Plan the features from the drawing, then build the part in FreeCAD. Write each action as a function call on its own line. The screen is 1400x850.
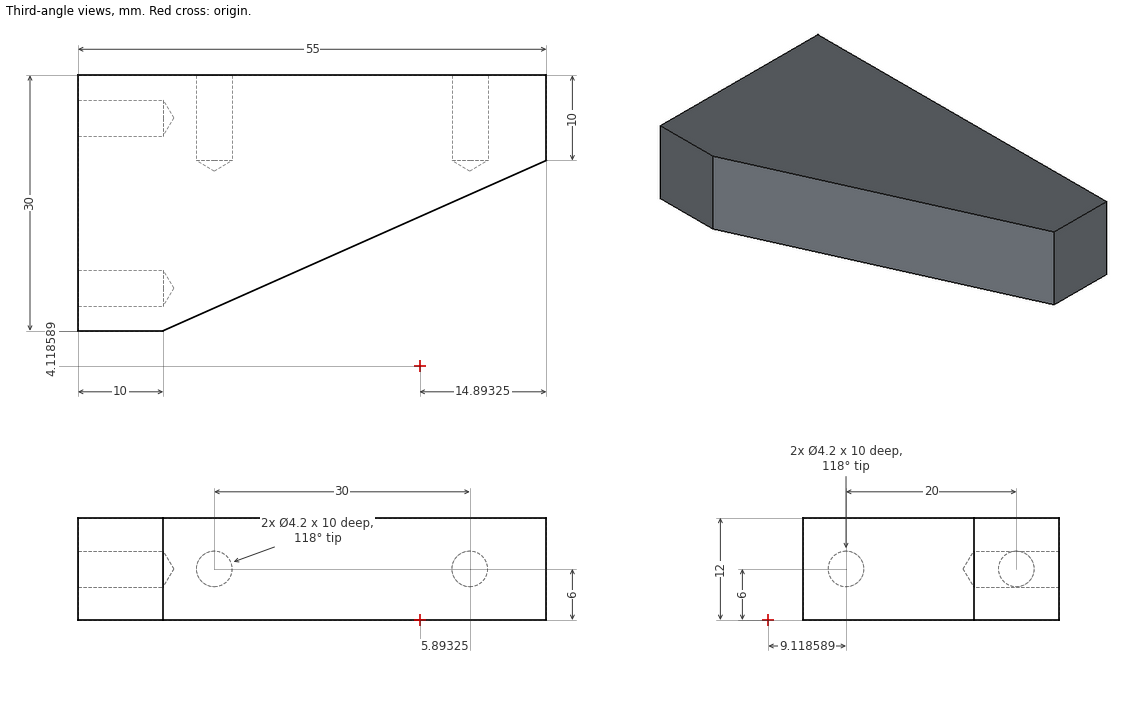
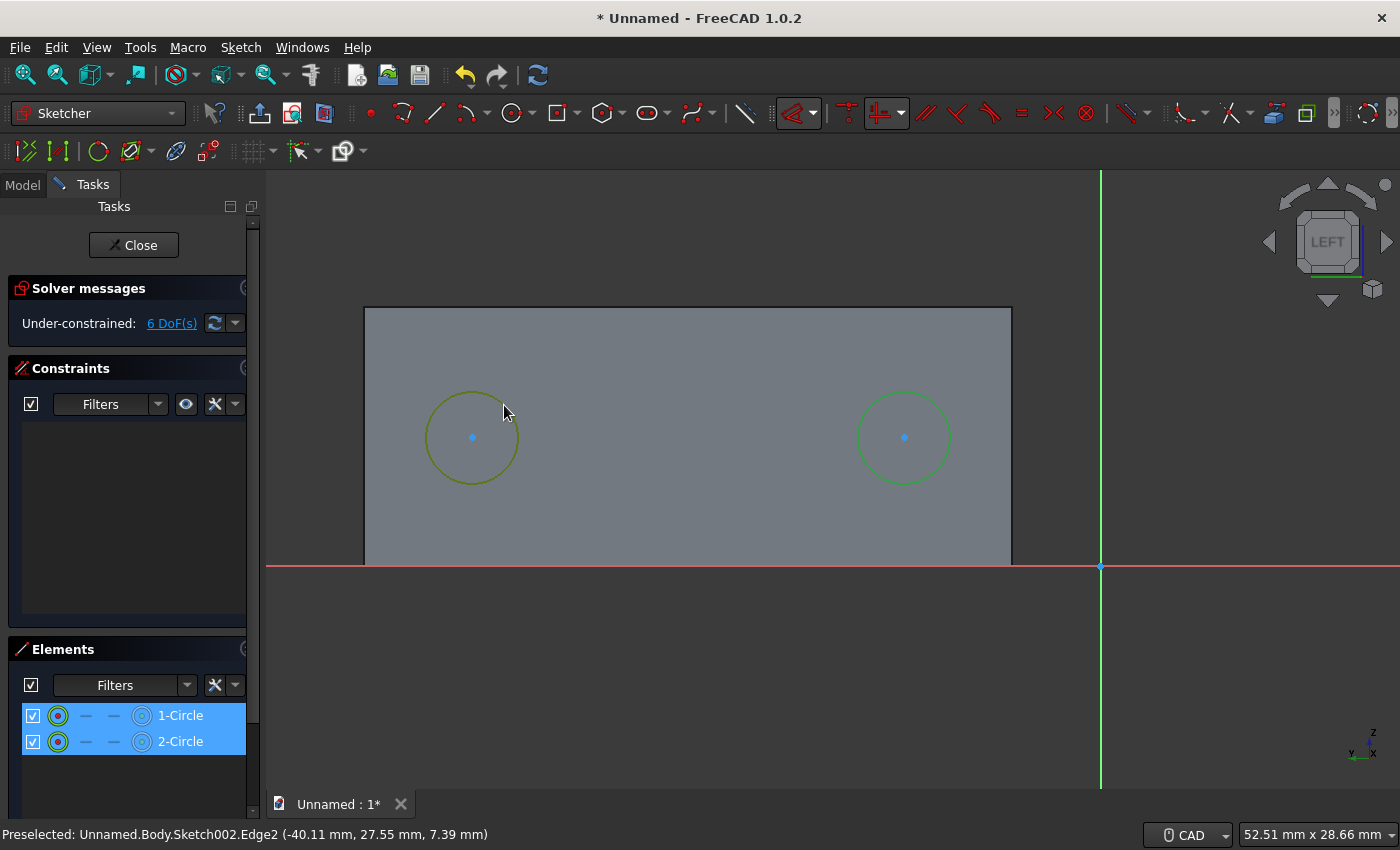
key(e)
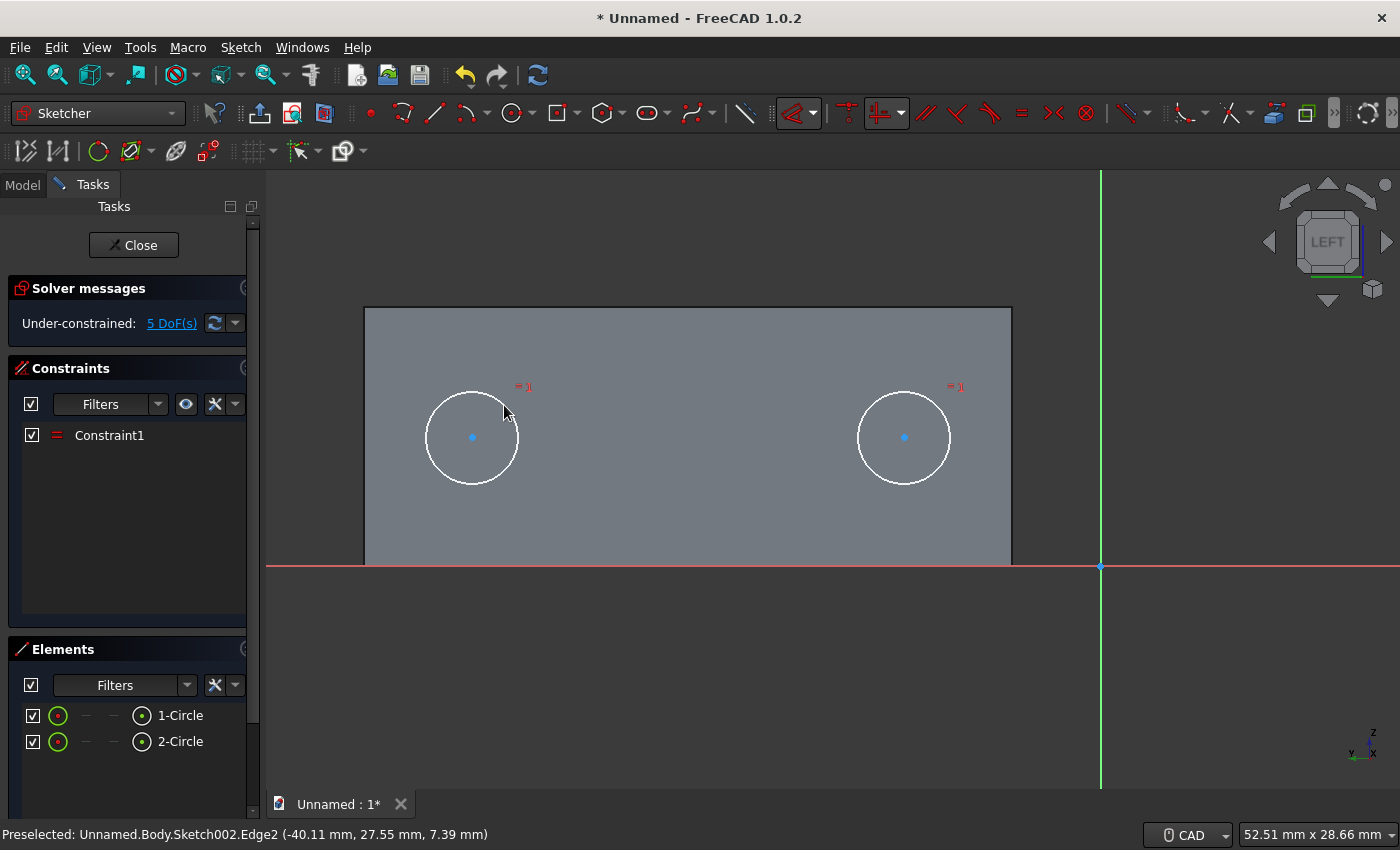
click(936, 405)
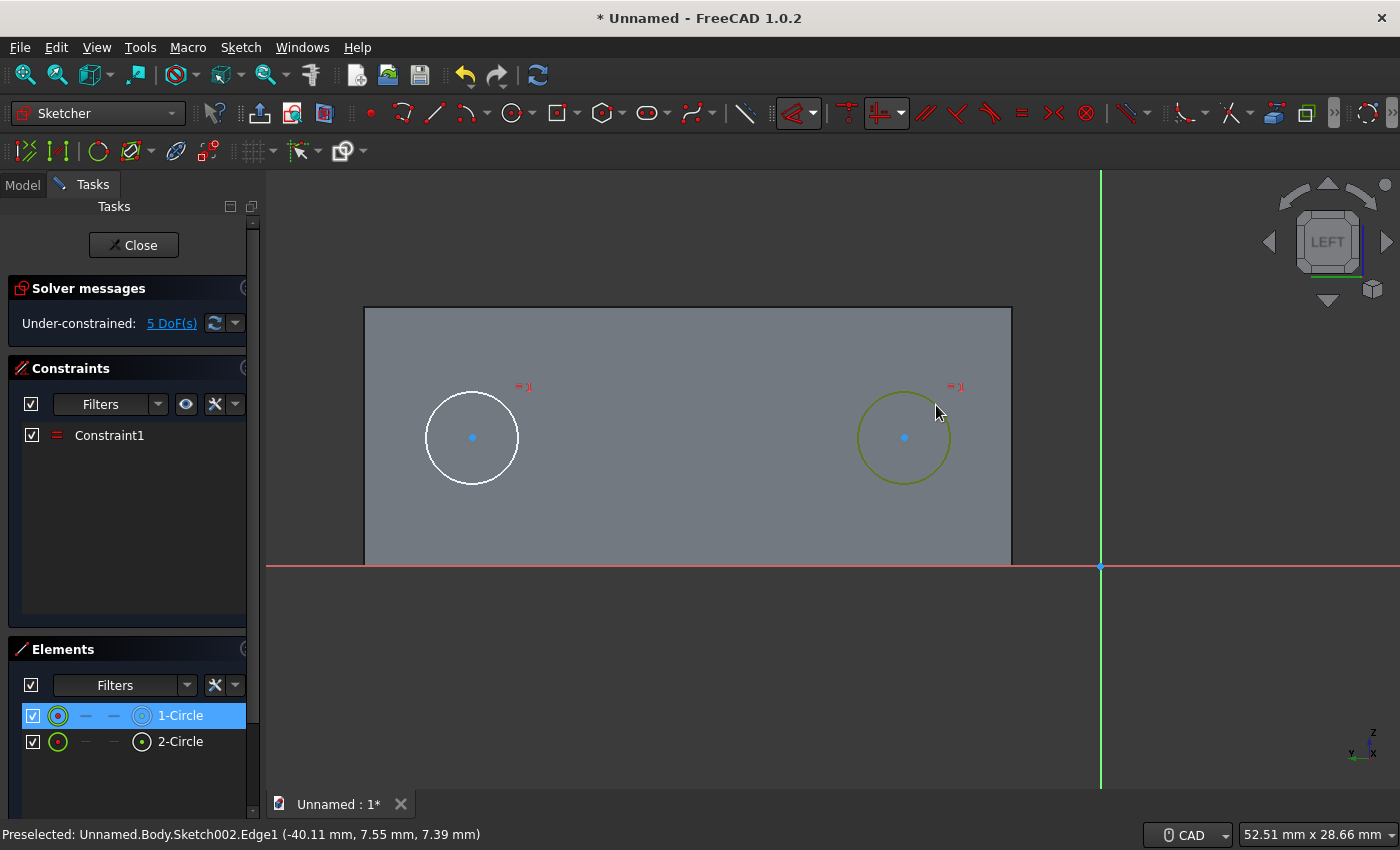
click(816, 114)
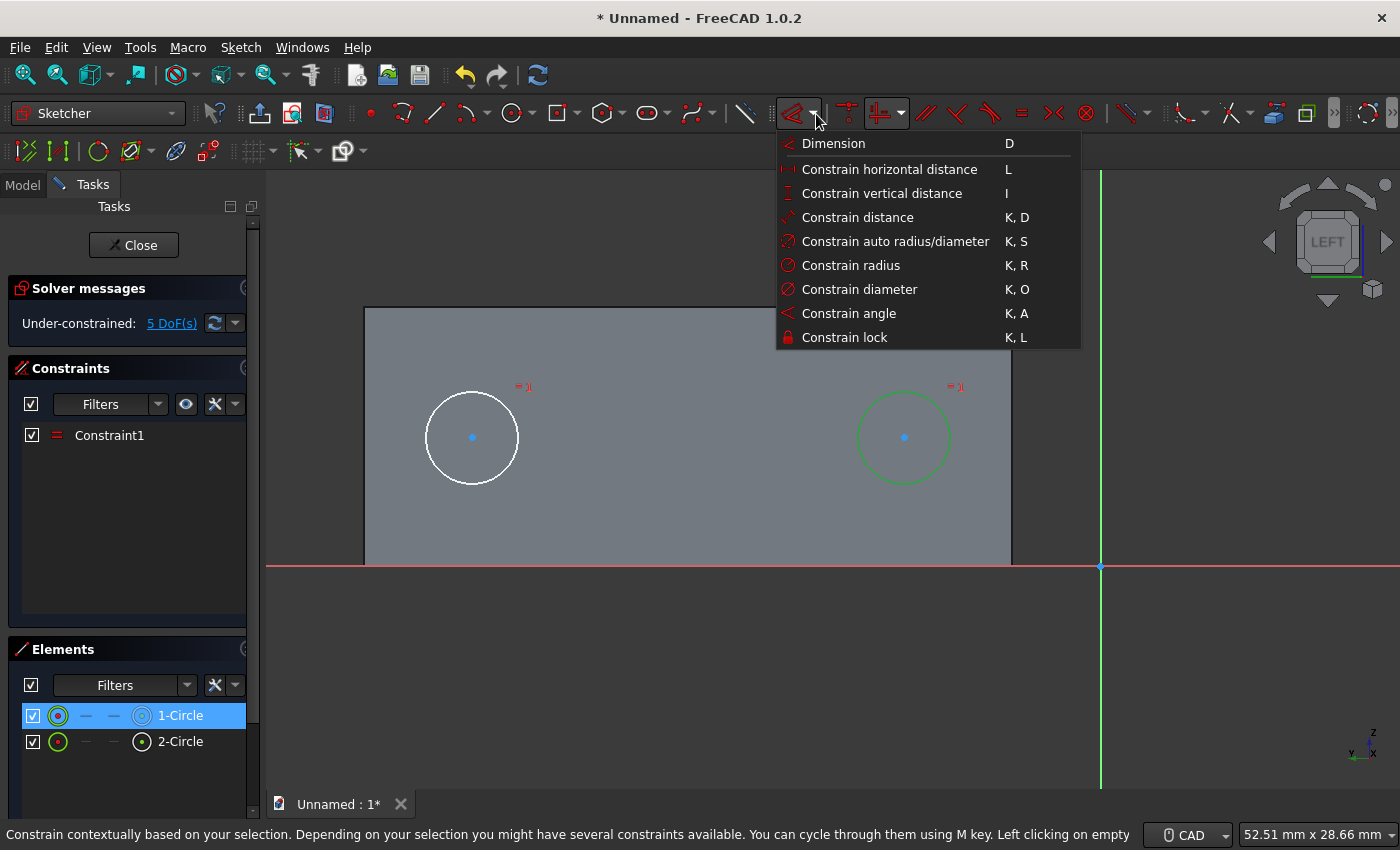
click(929, 289)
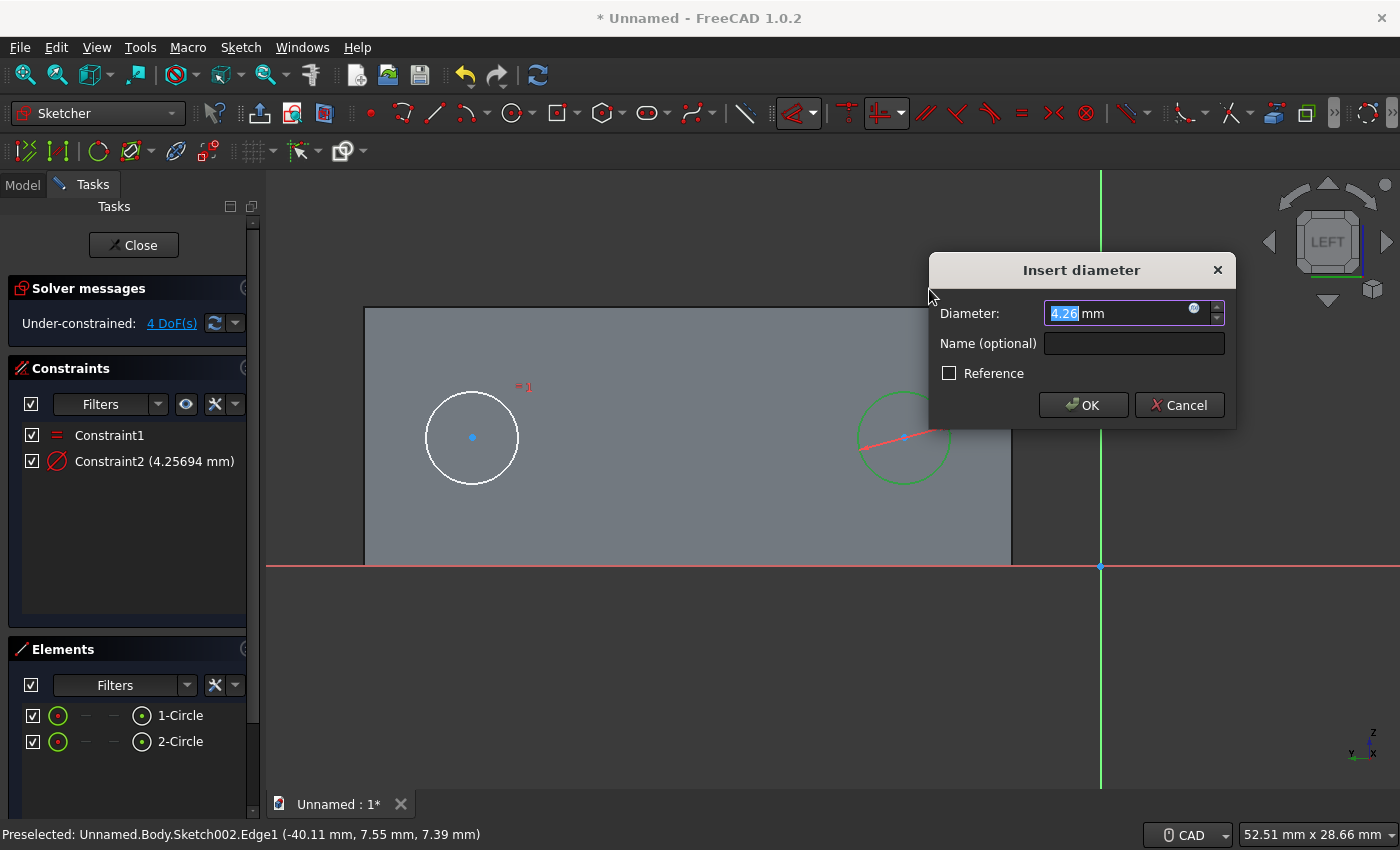
text(4.2)
key(Return)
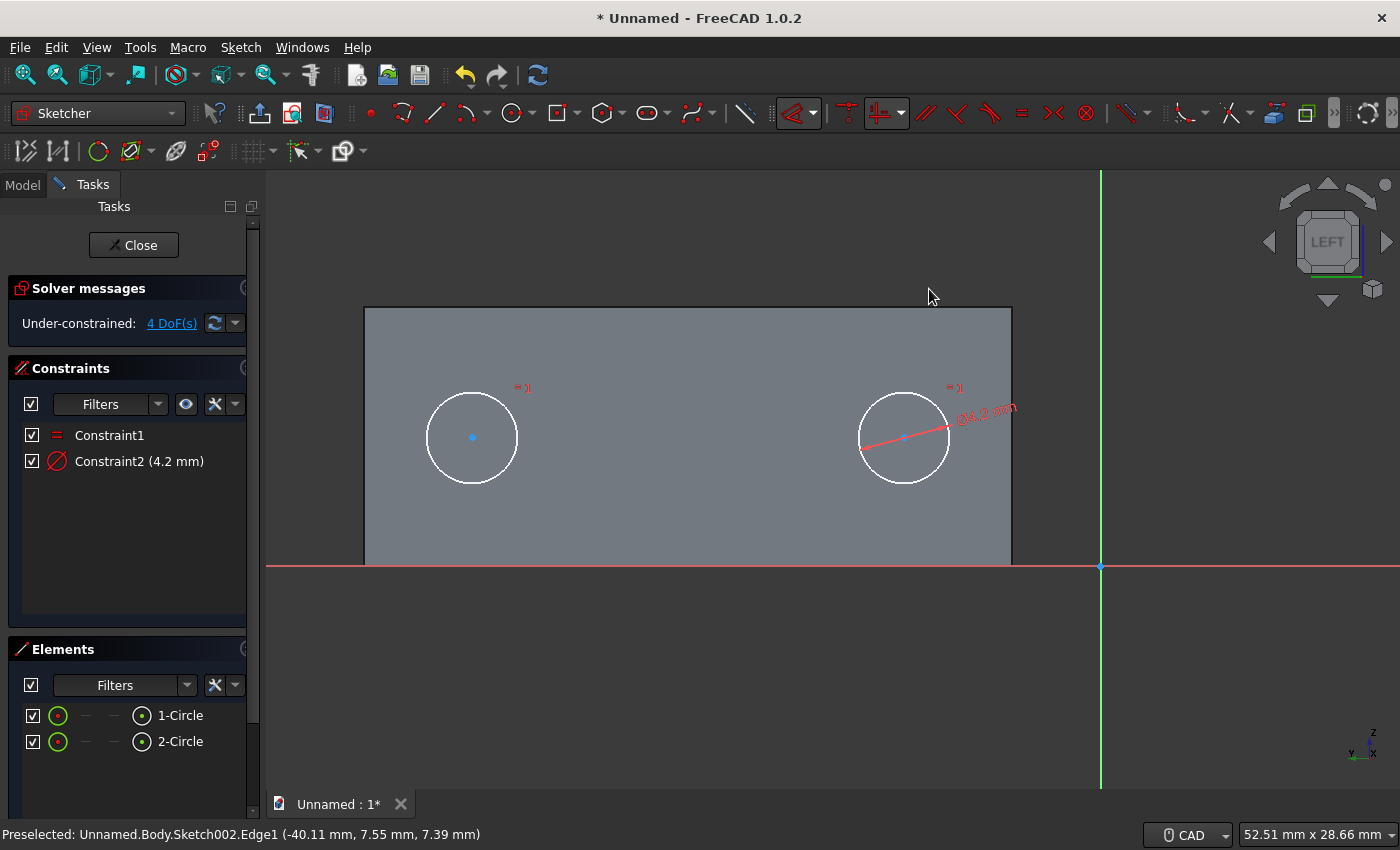
click(904, 438)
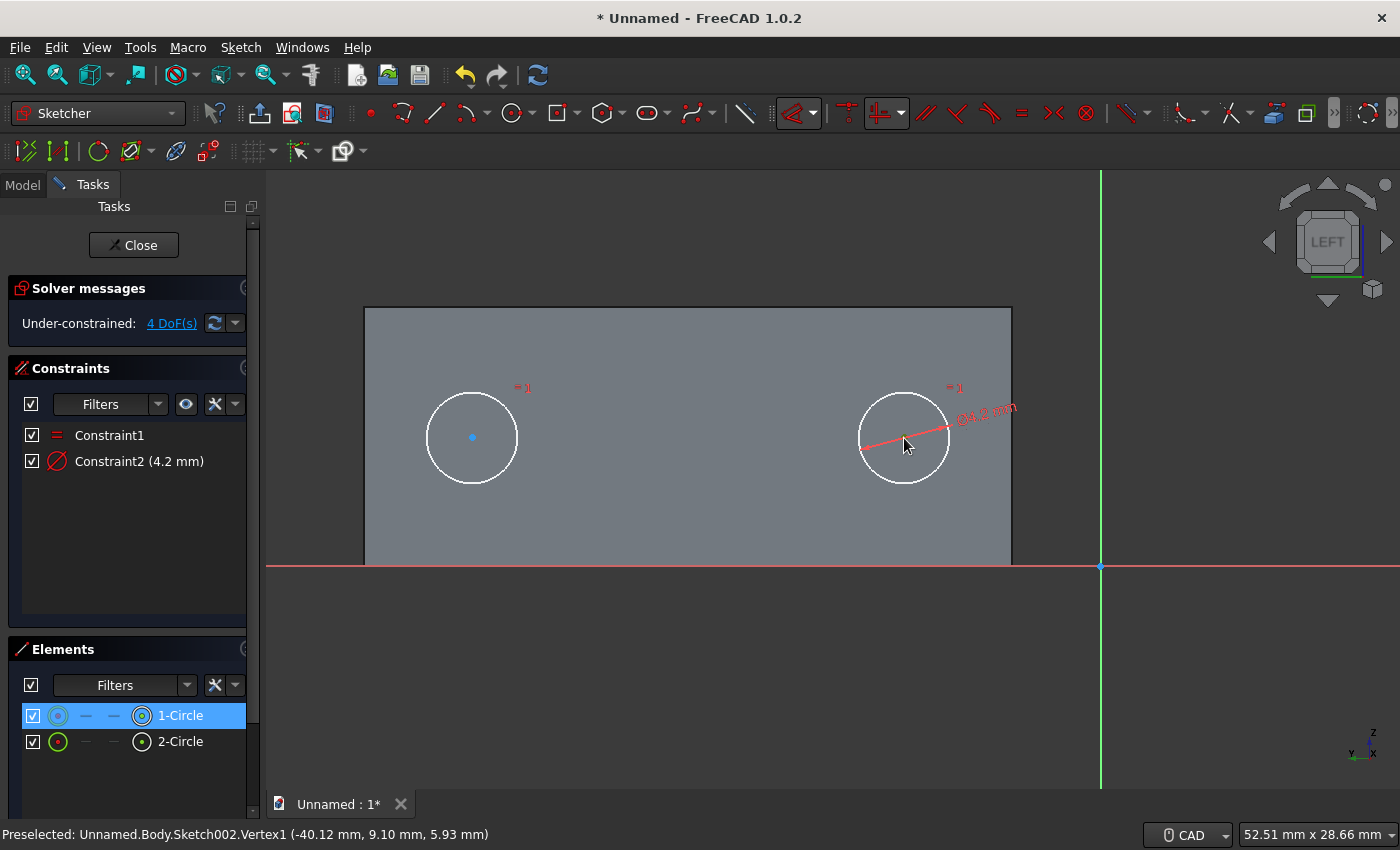
key(i)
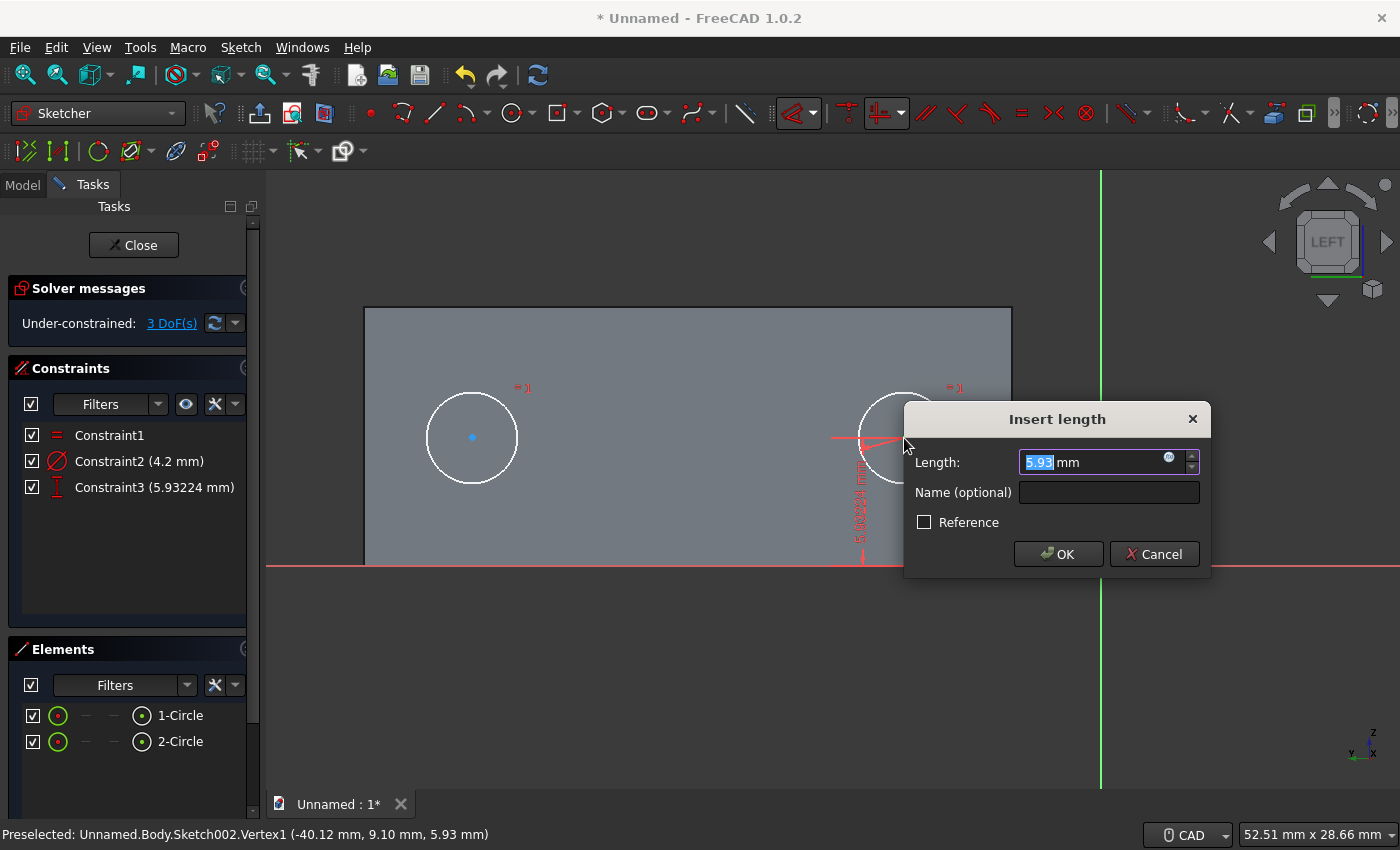
text(6)
key(Return)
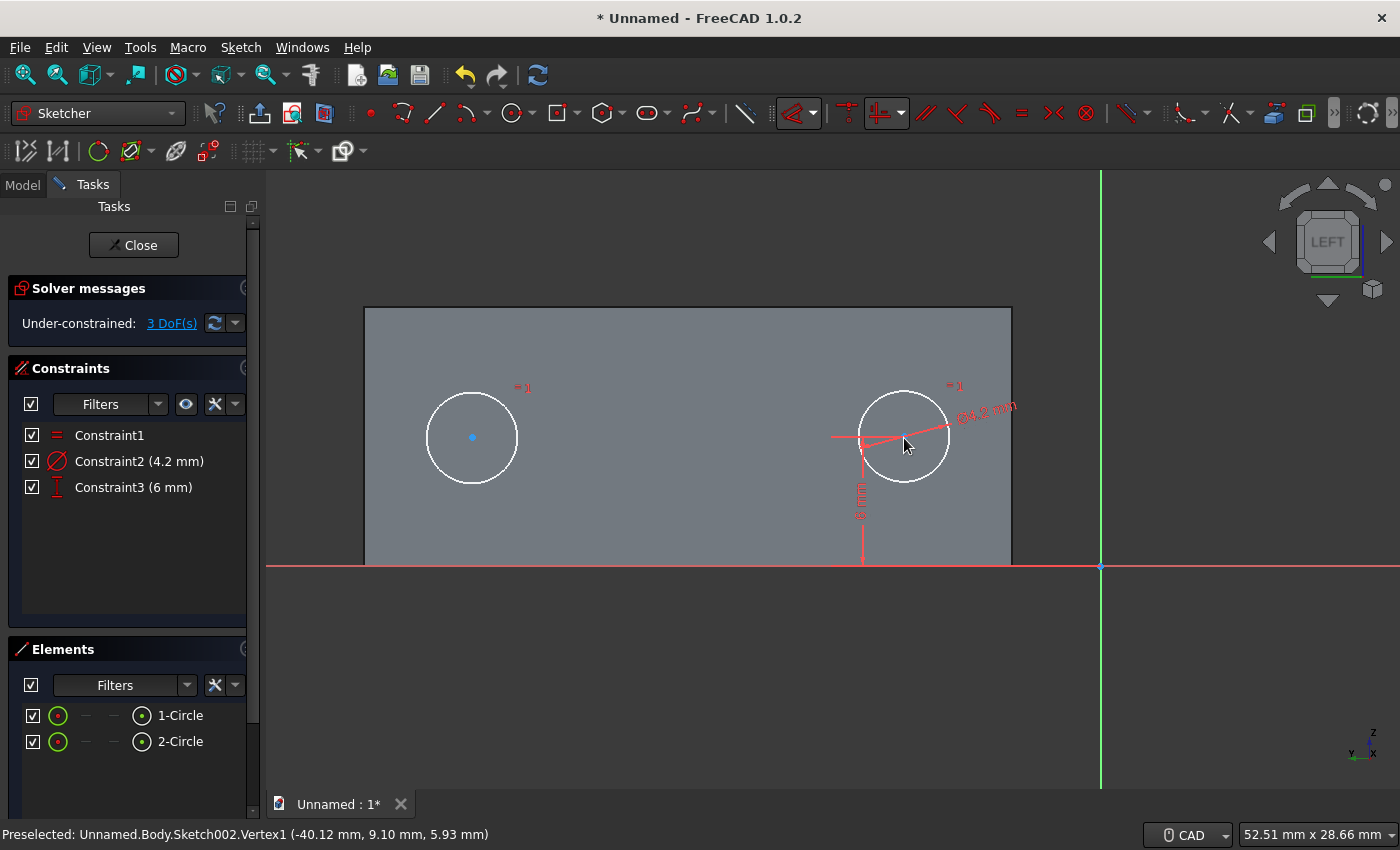
click(472, 438)